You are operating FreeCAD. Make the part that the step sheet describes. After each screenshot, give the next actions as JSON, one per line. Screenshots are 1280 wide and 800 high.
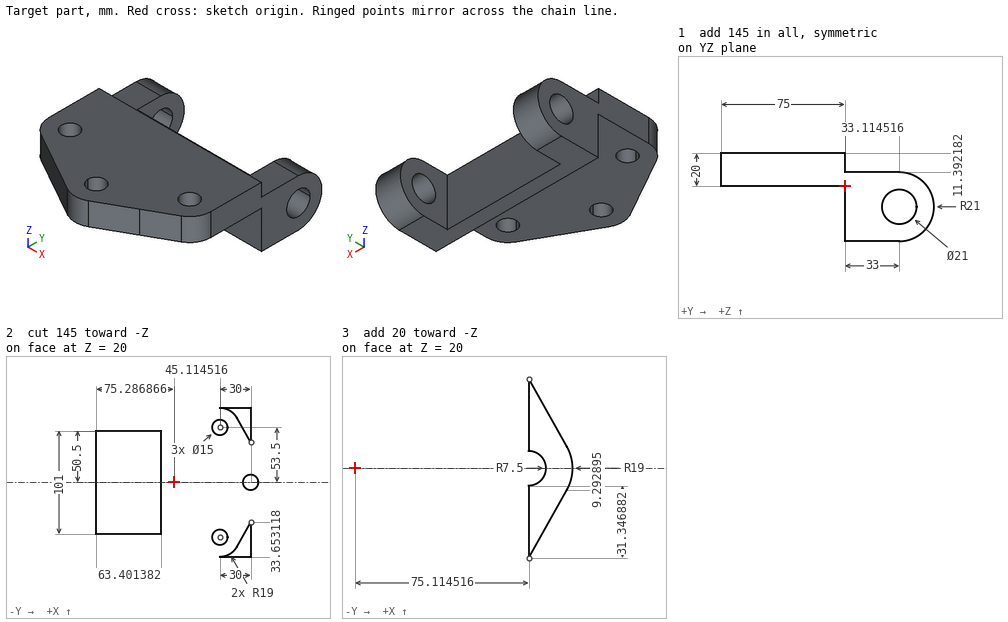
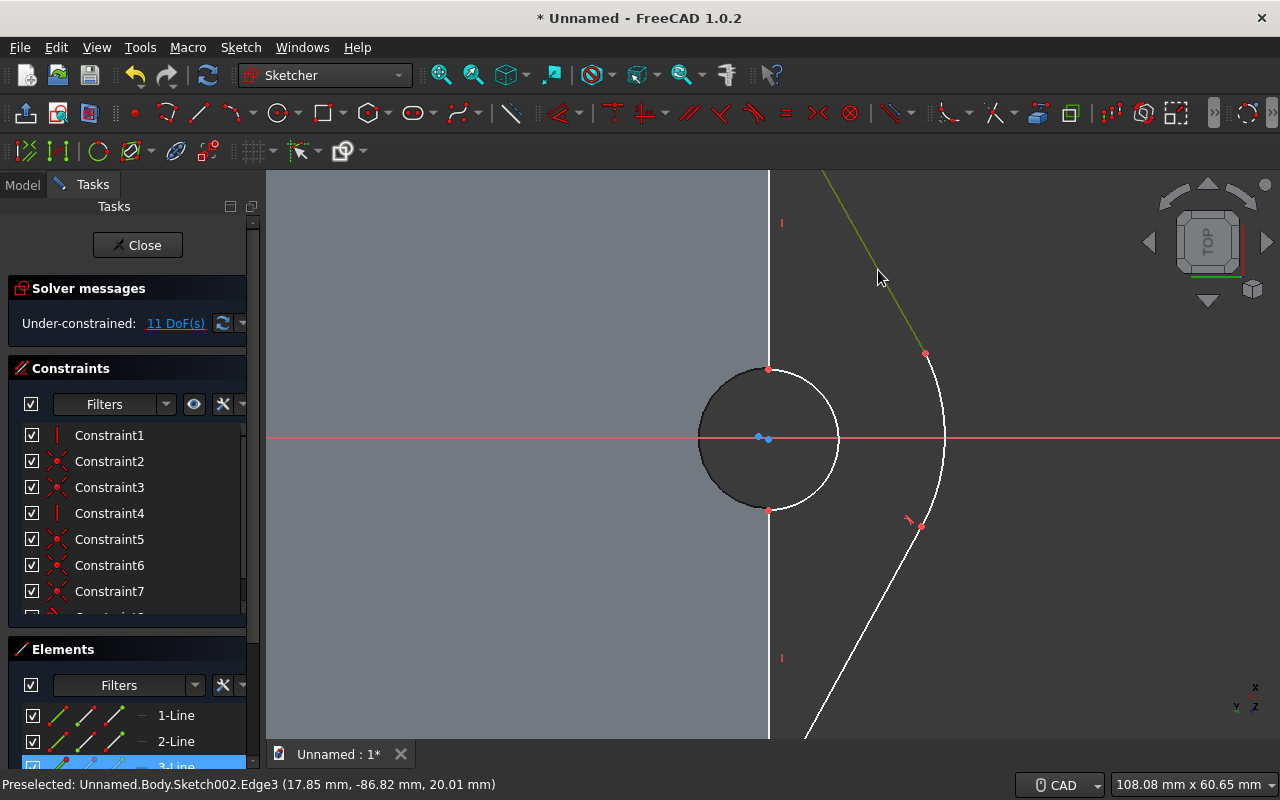
{"action": "left_click", "coordinate": [941, 476]}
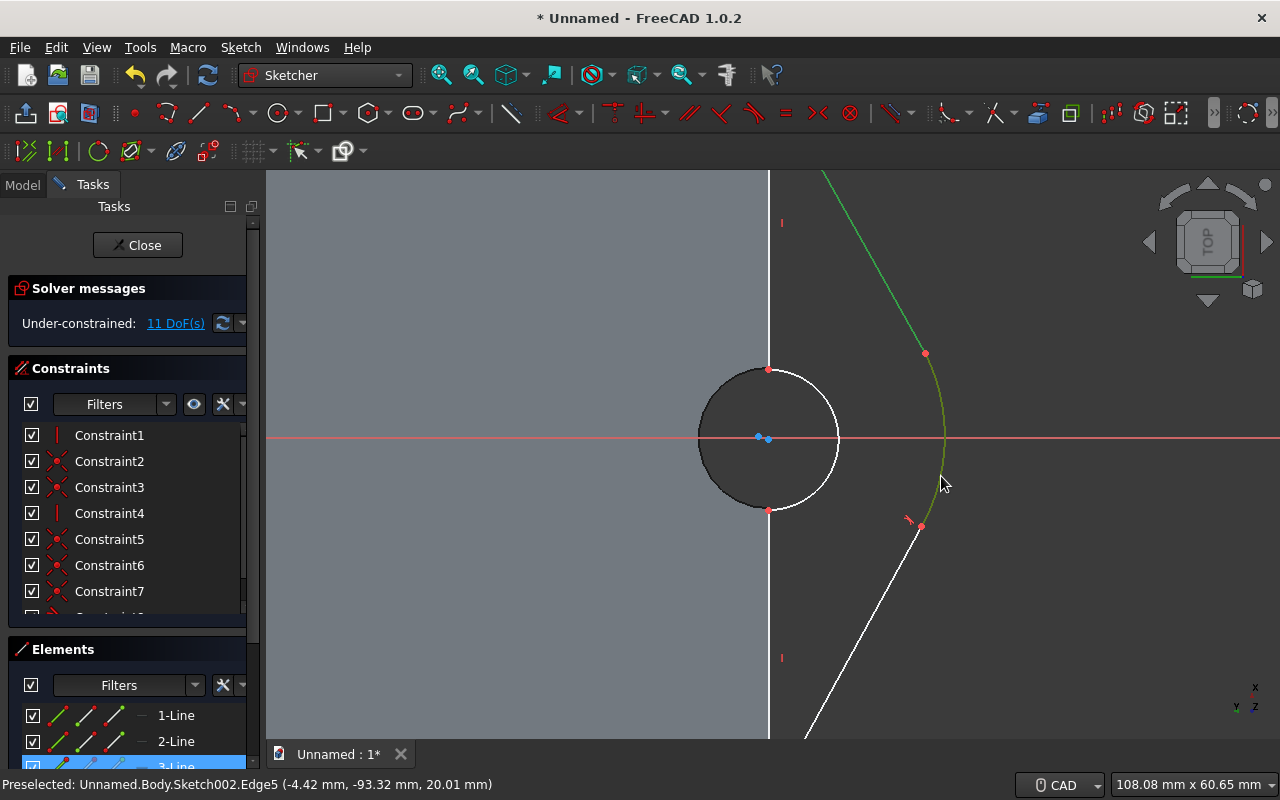
{"action": "left_click", "coordinate": [754, 114]}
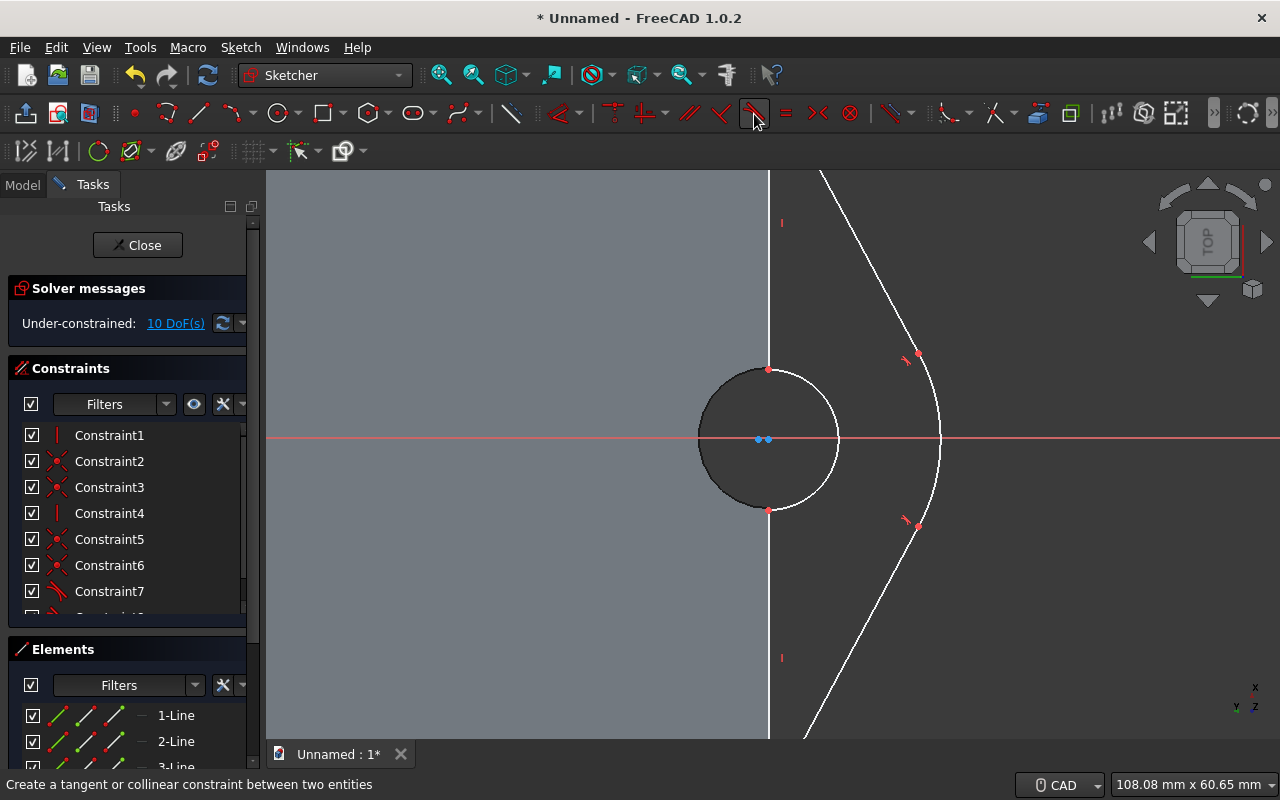
{"action": "left_click", "coordinate": [937, 476]}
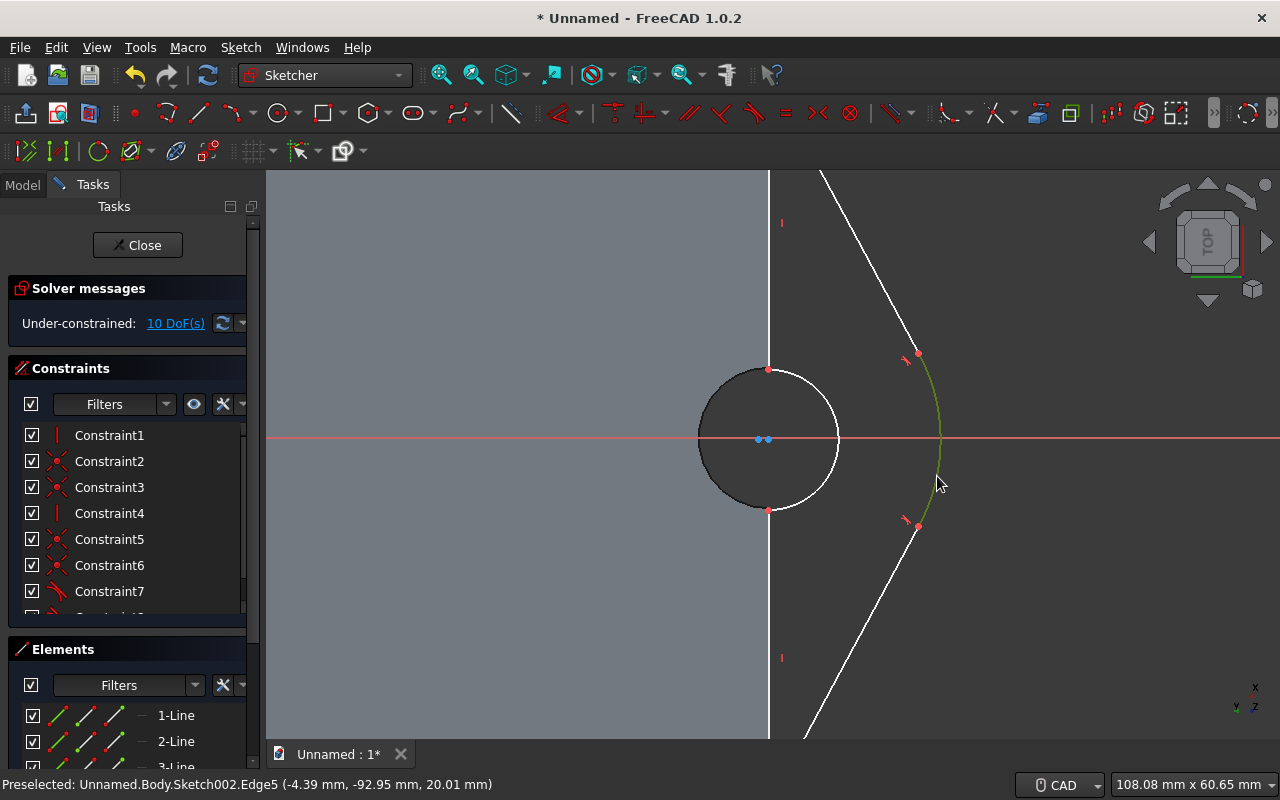
{"action": "left_click", "coordinate": [825, 481]}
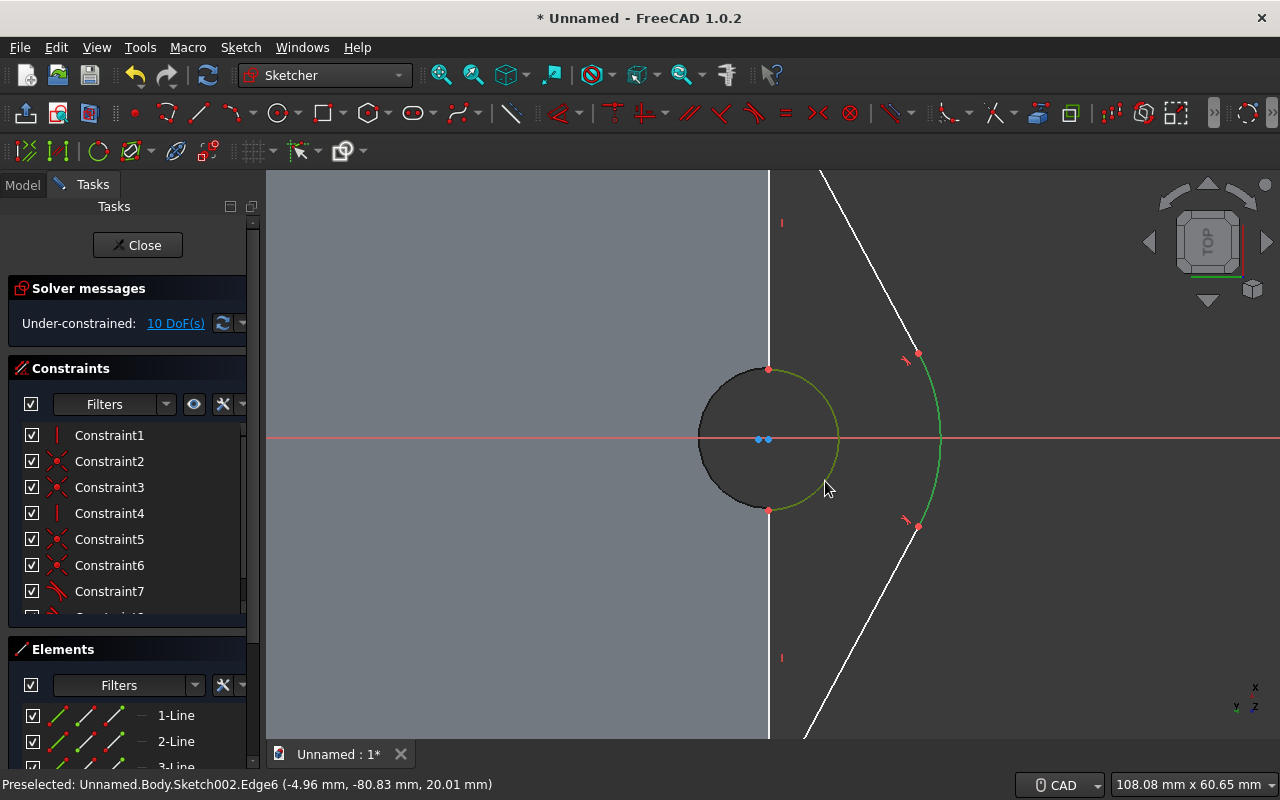
{"action": "left_click", "coordinate": [614, 114]}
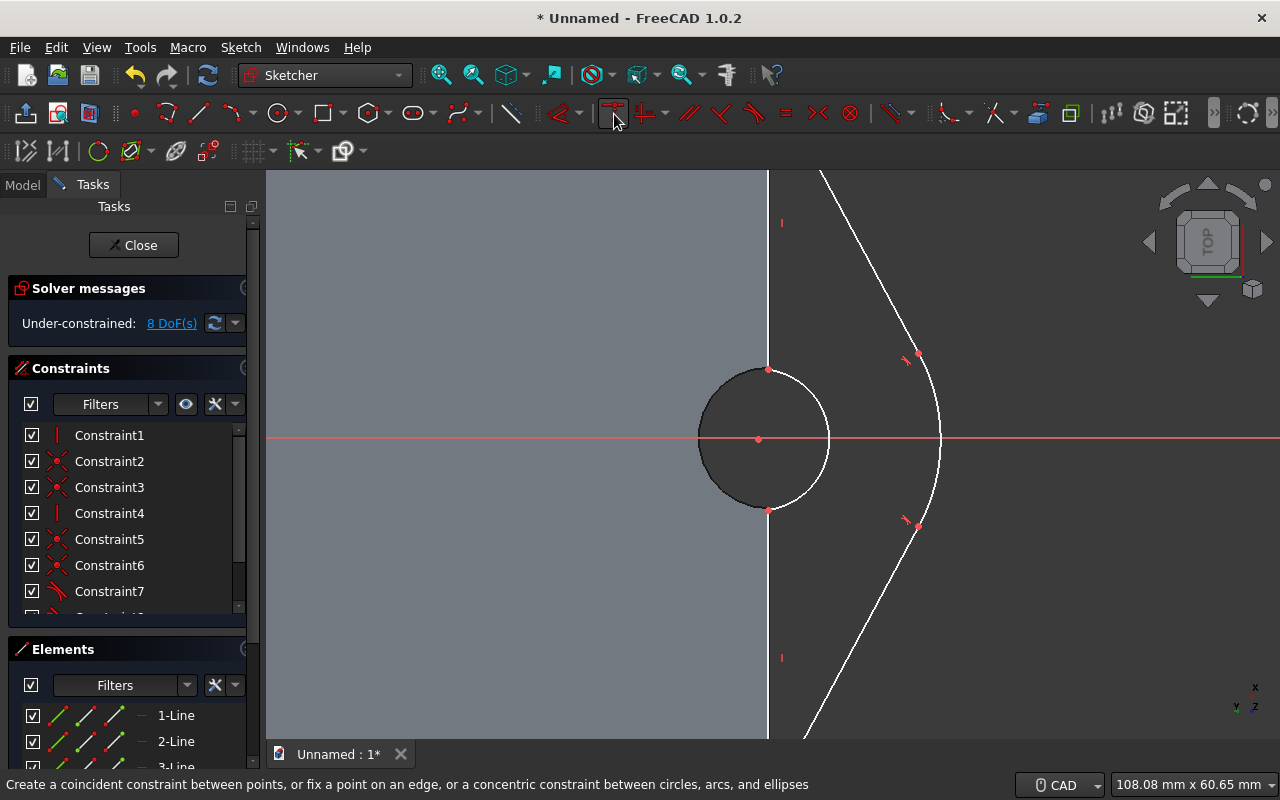
{"action": "left_click", "coordinate": [758, 440]}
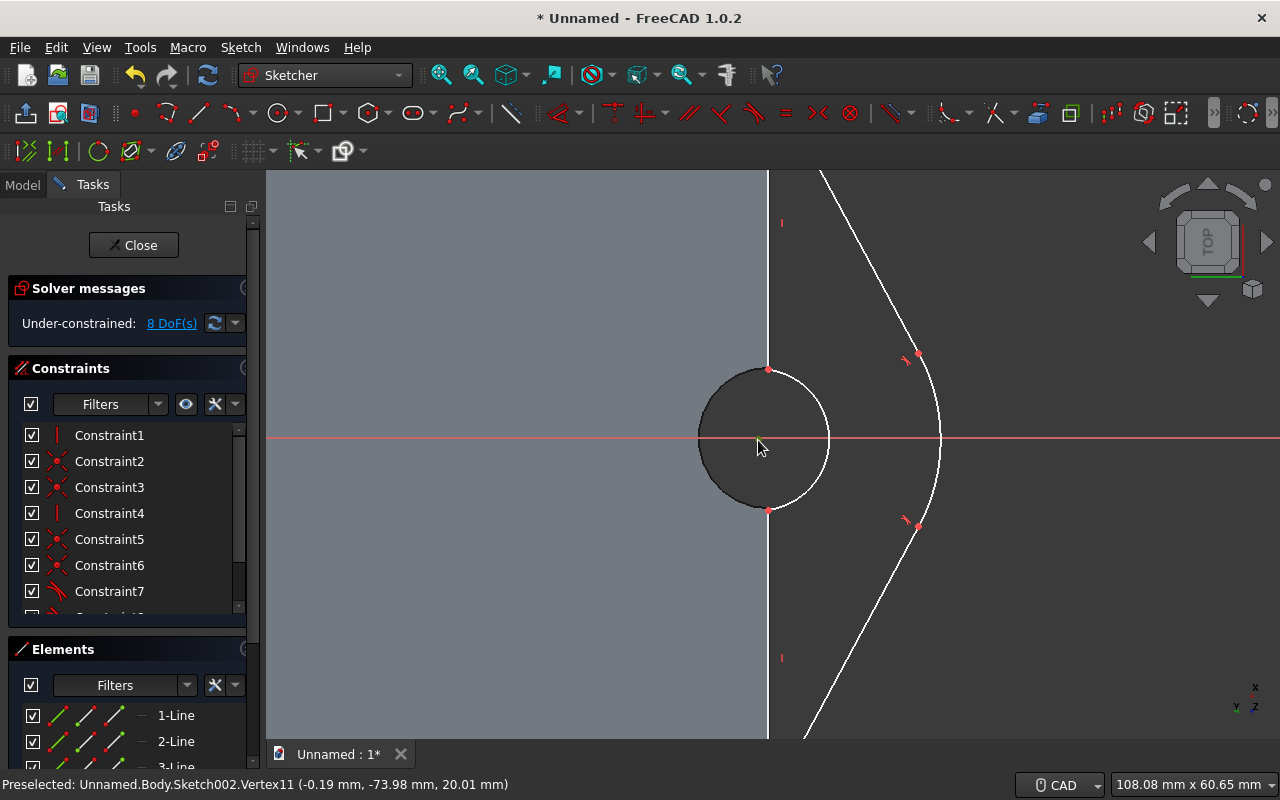
{"action": "left_click", "coordinate": [353, 438]}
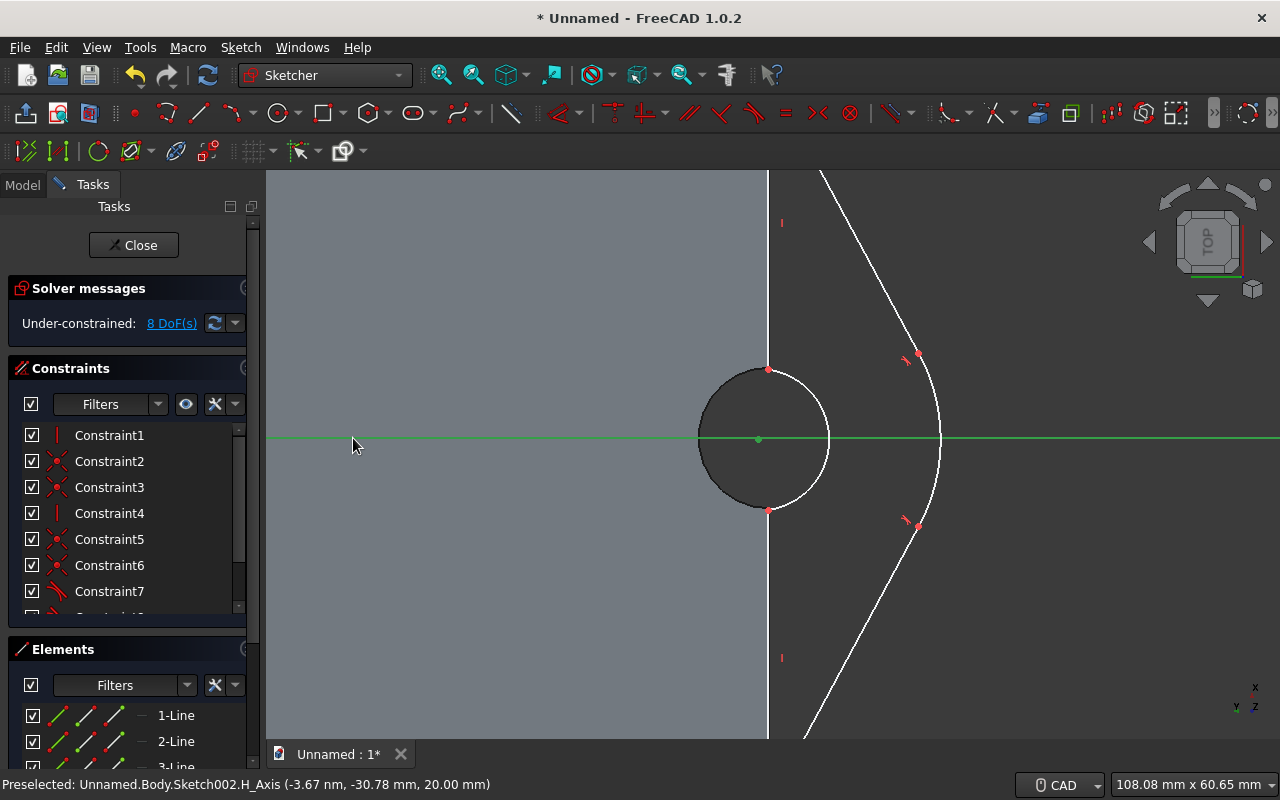
{"action": "left_click", "coordinate": [614, 114]}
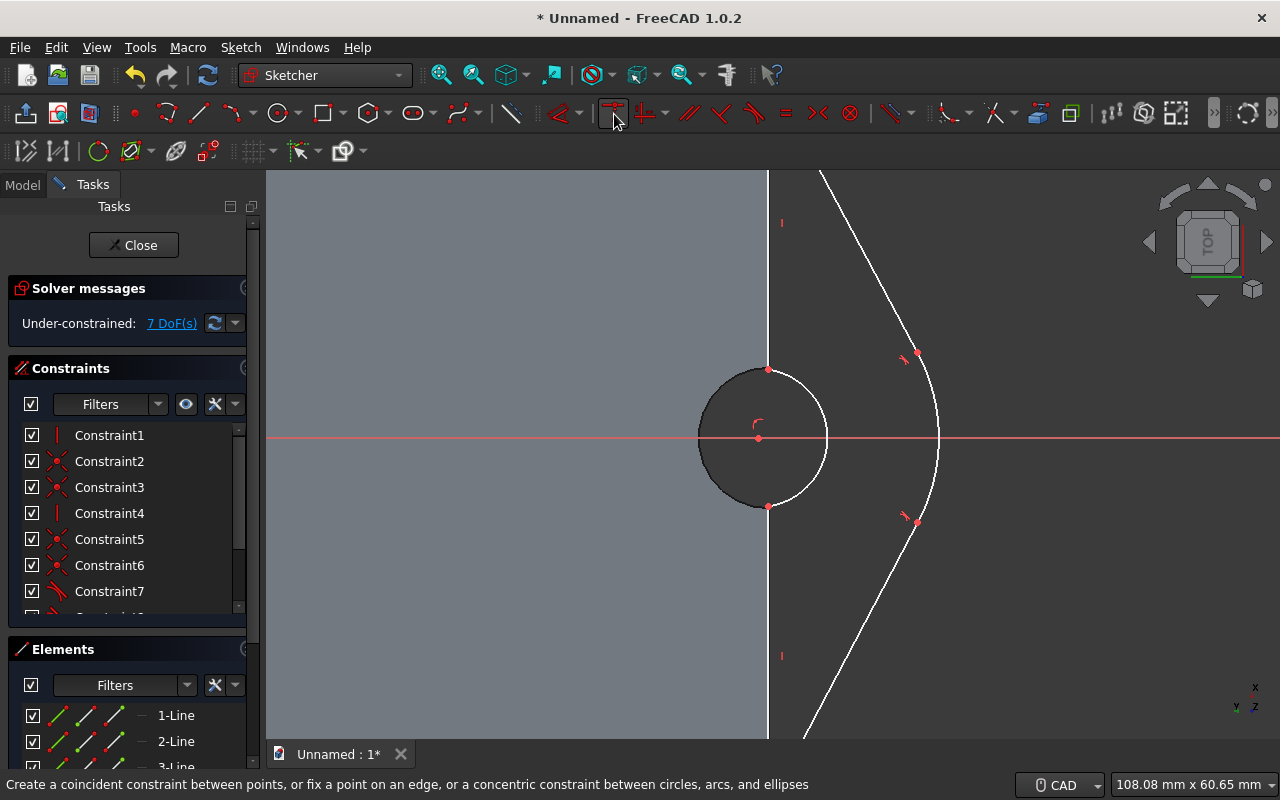
{"action": "scroll", "coordinate": [946, 475], "scroll_direction": "down", "scroll_amount": 3}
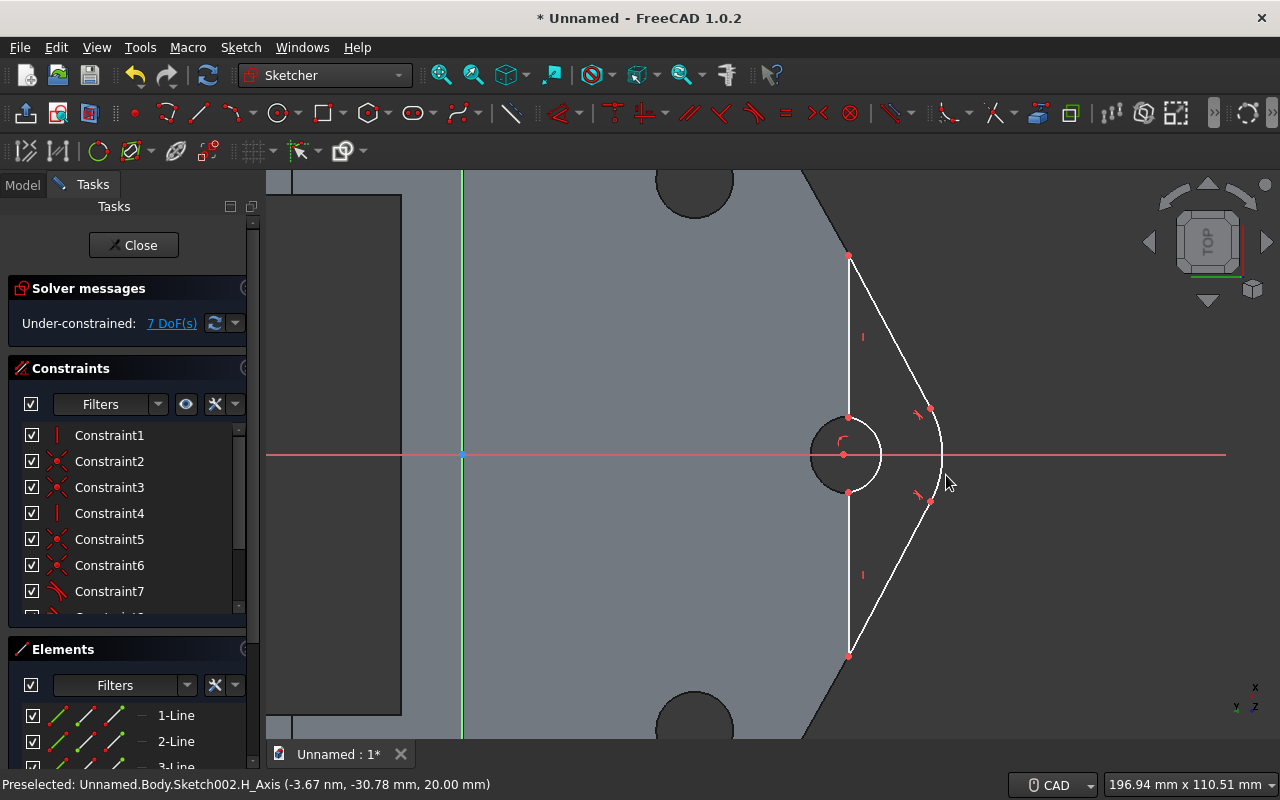
{"action": "left_click", "coordinate": [849, 656]}